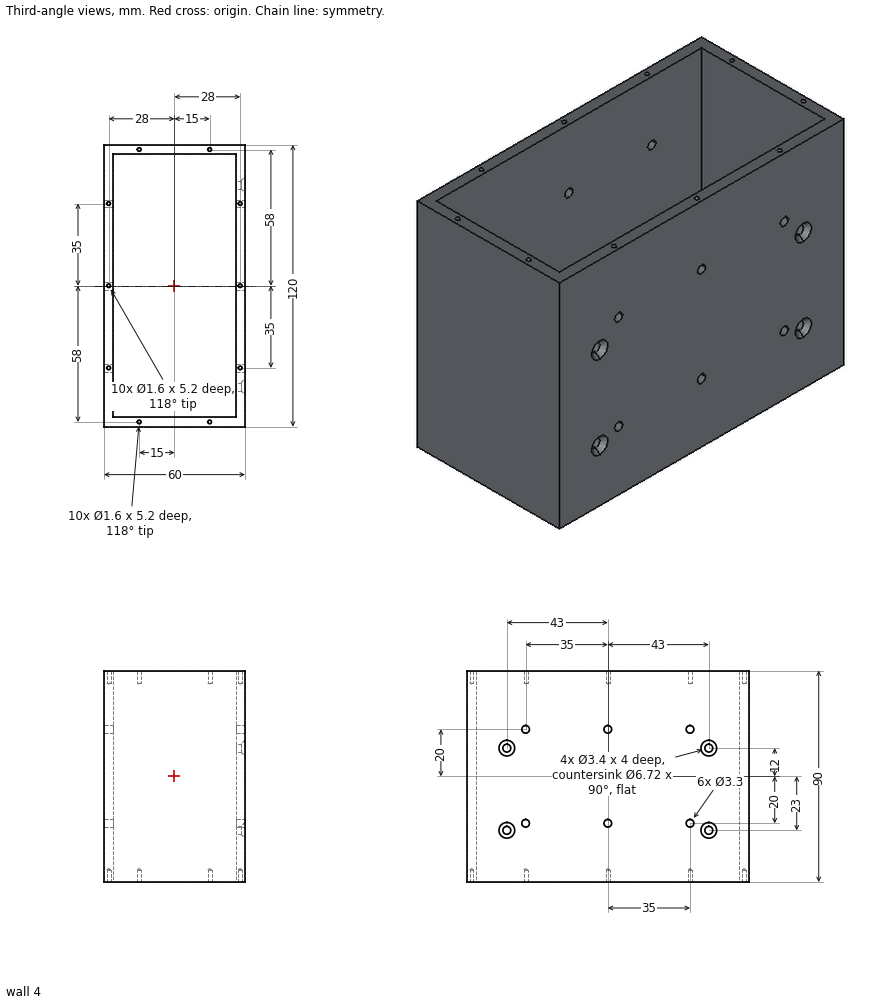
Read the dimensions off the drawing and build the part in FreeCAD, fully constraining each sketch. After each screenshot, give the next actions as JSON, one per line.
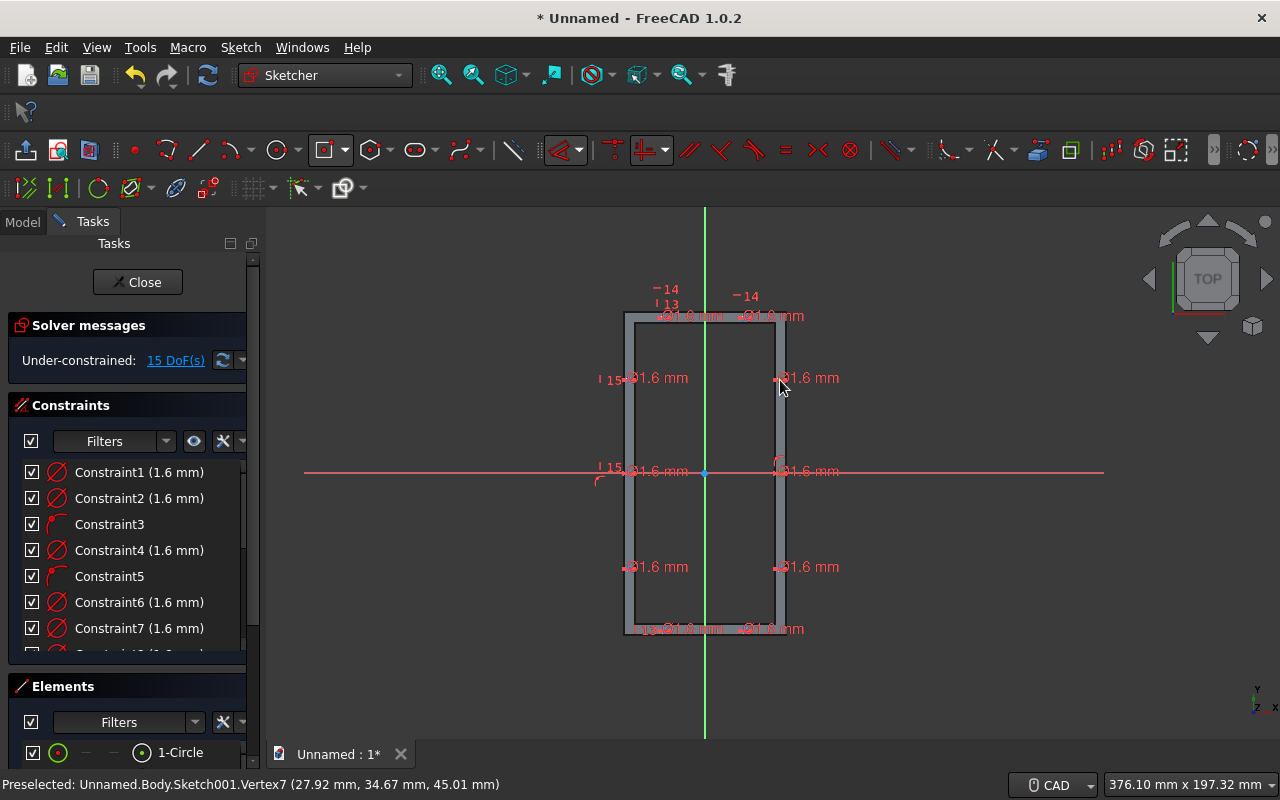
{"action": "left_click", "coordinate": [668, 150]}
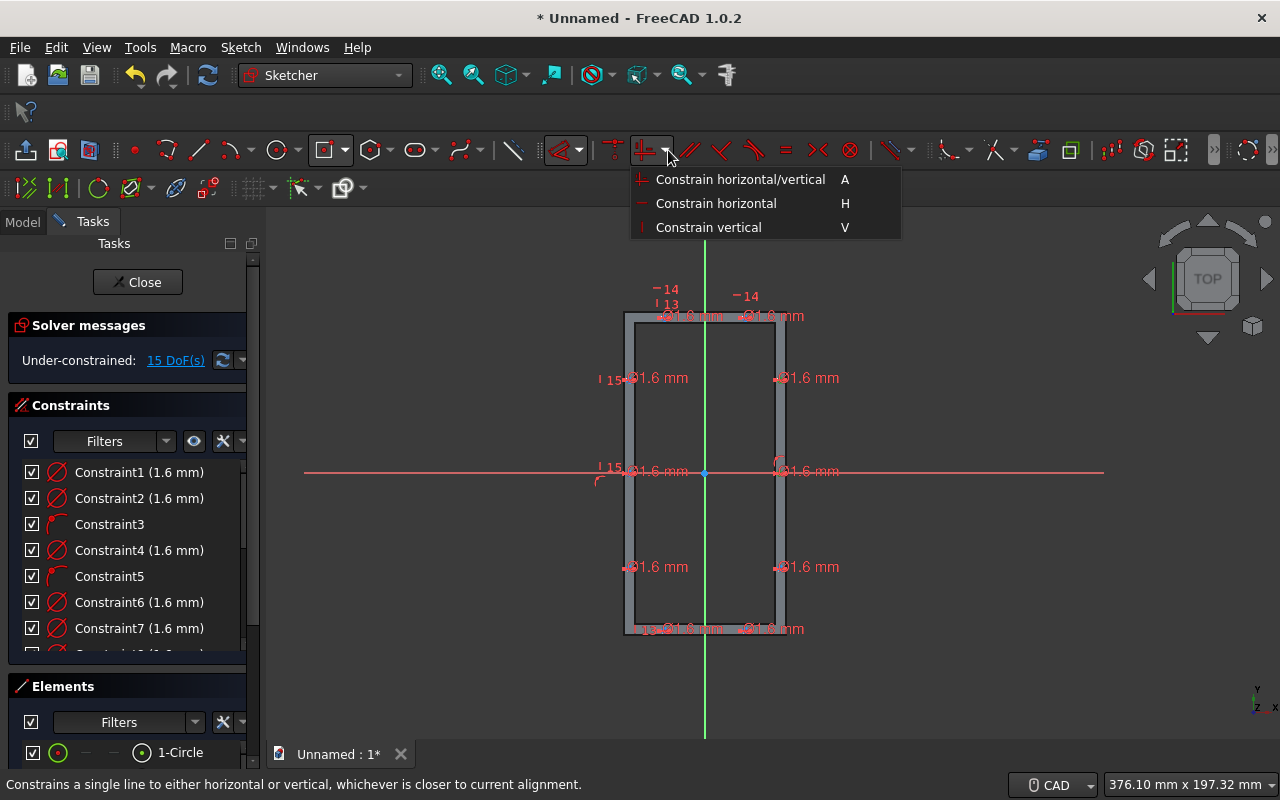
{"action": "left_click", "coordinate": [766, 227]}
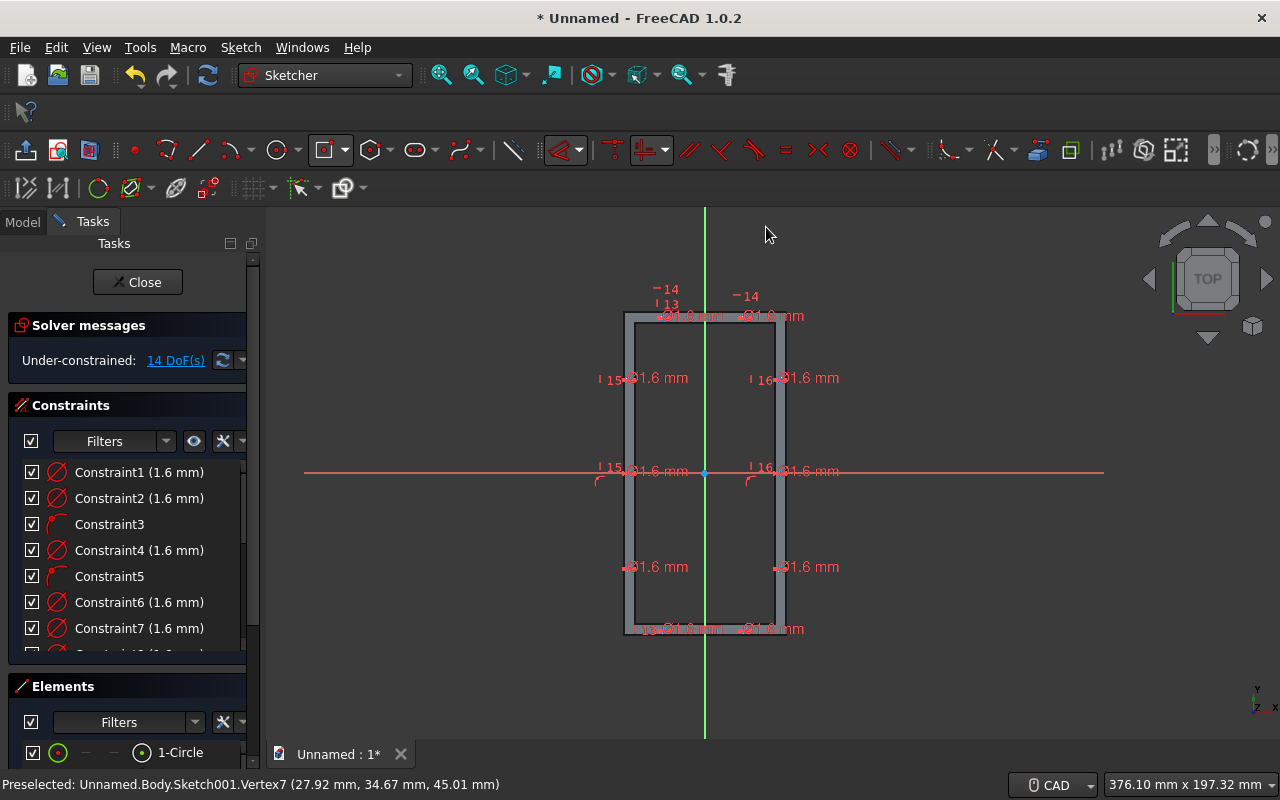
{"action": "left_click", "coordinate": [629, 380]}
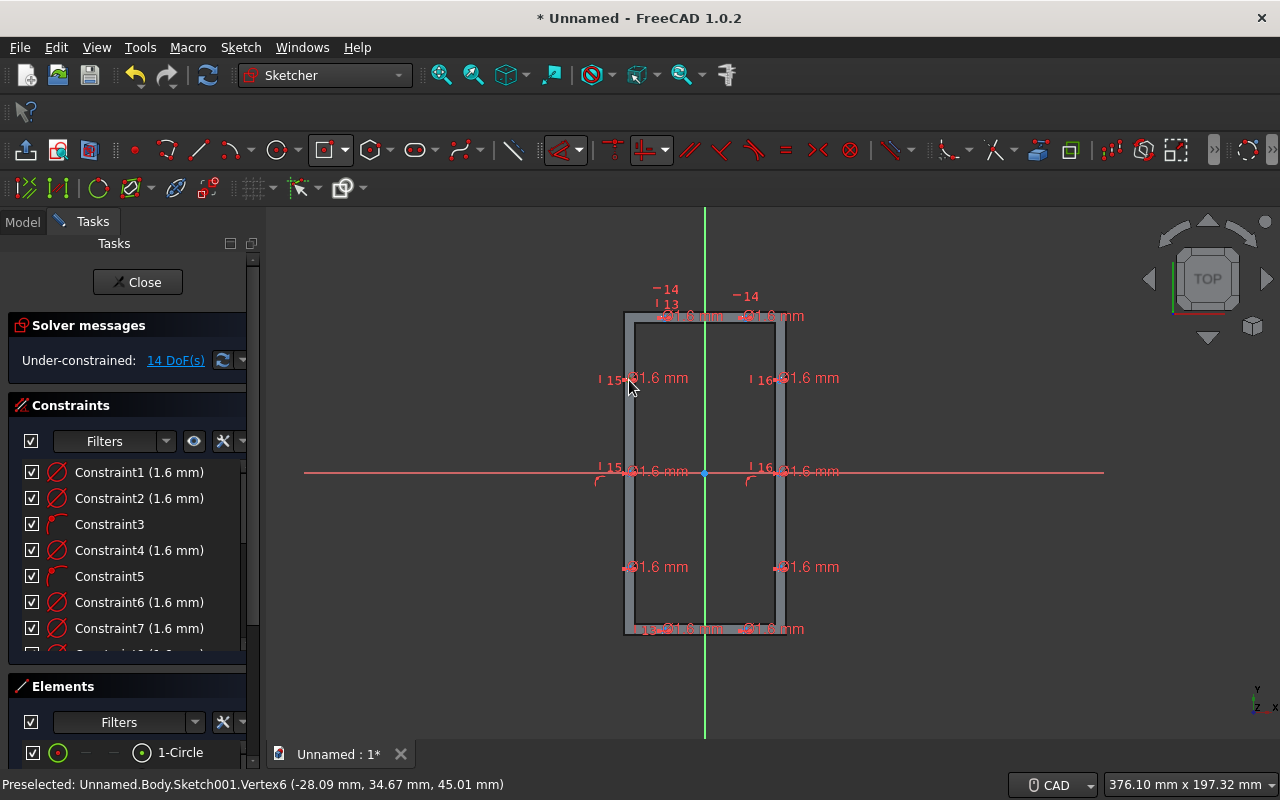
{"action": "left_click", "coordinate": [780, 380]}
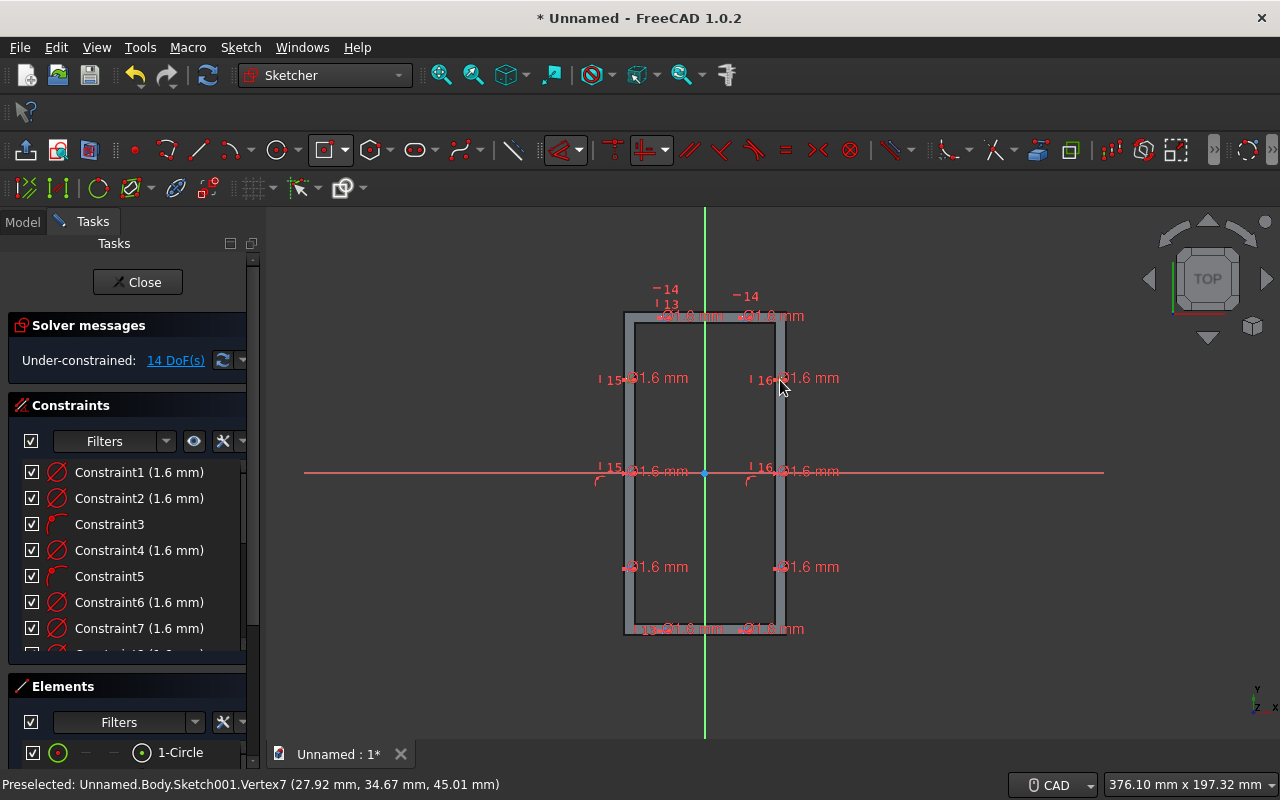
{"action": "left_click", "coordinate": [668, 150]}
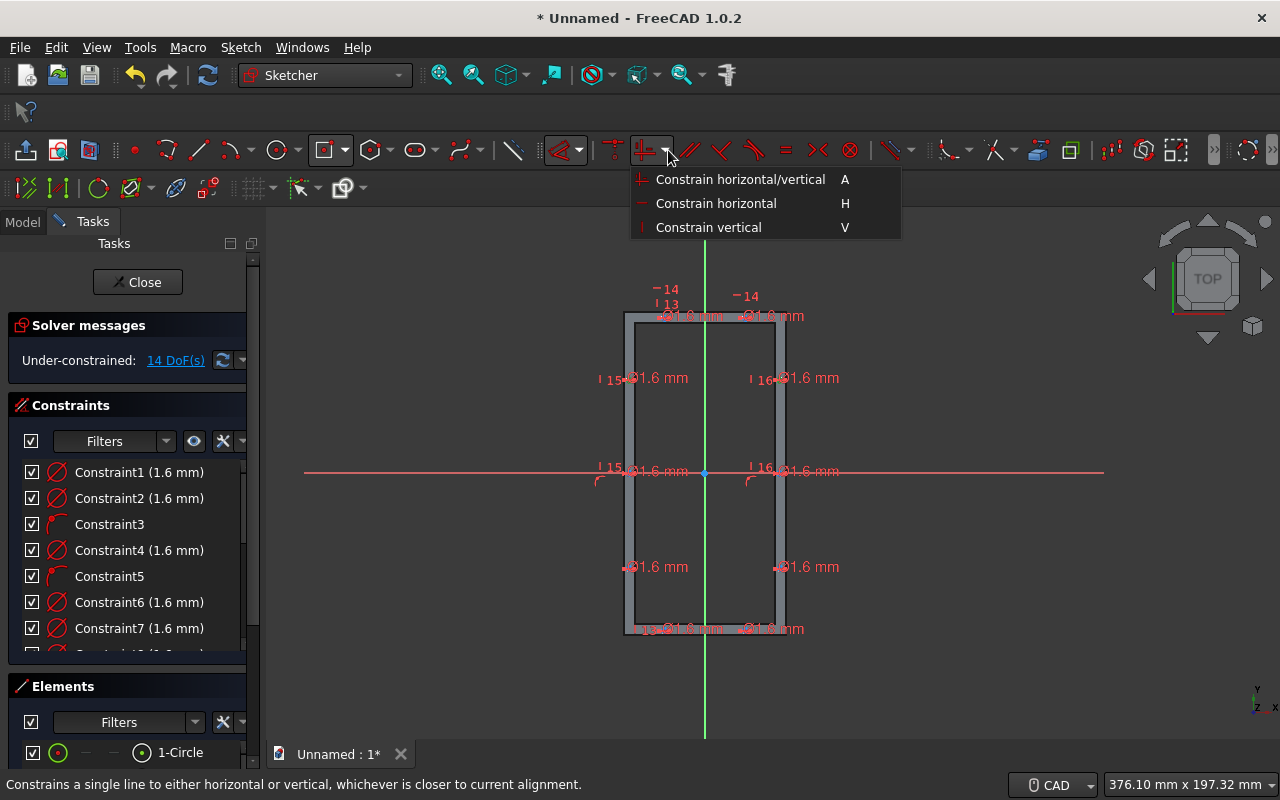
{"action": "left_click", "coordinate": [766, 203]}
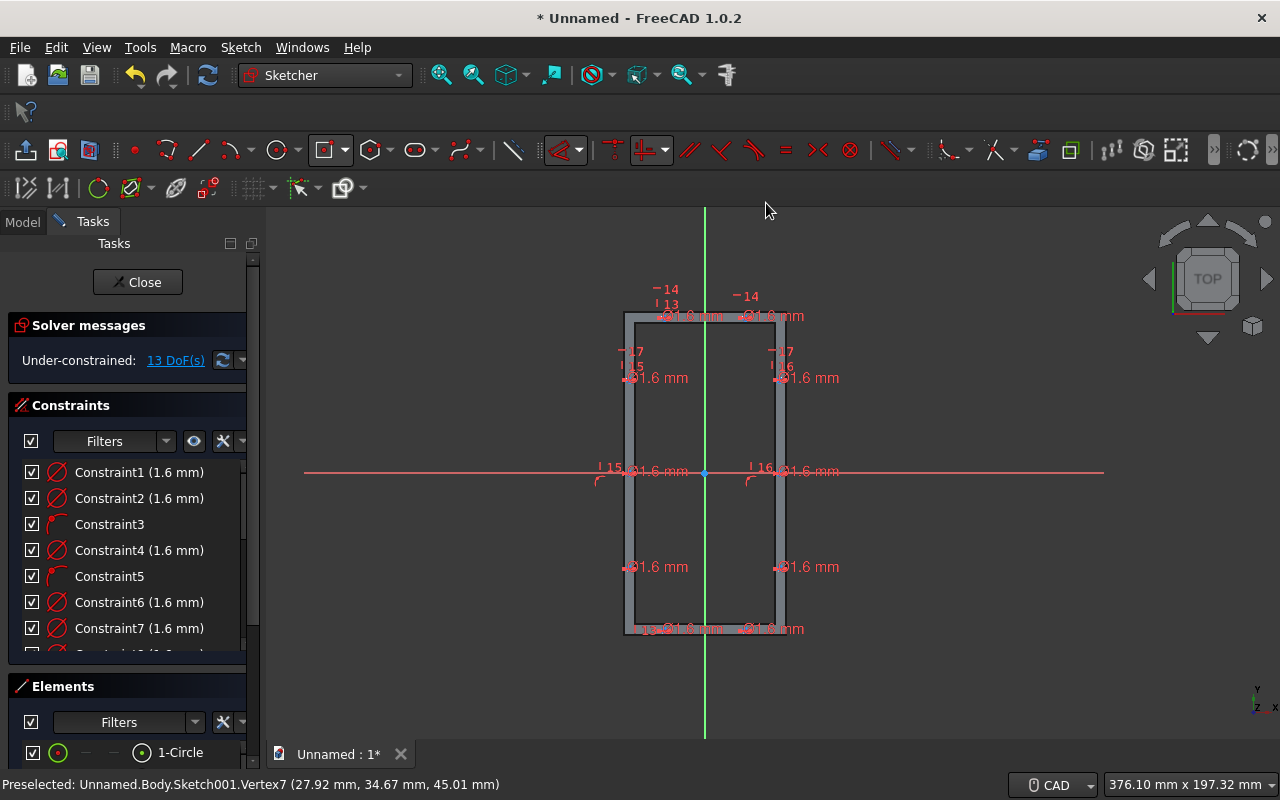
{"action": "left_click", "coordinate": [780, 473]}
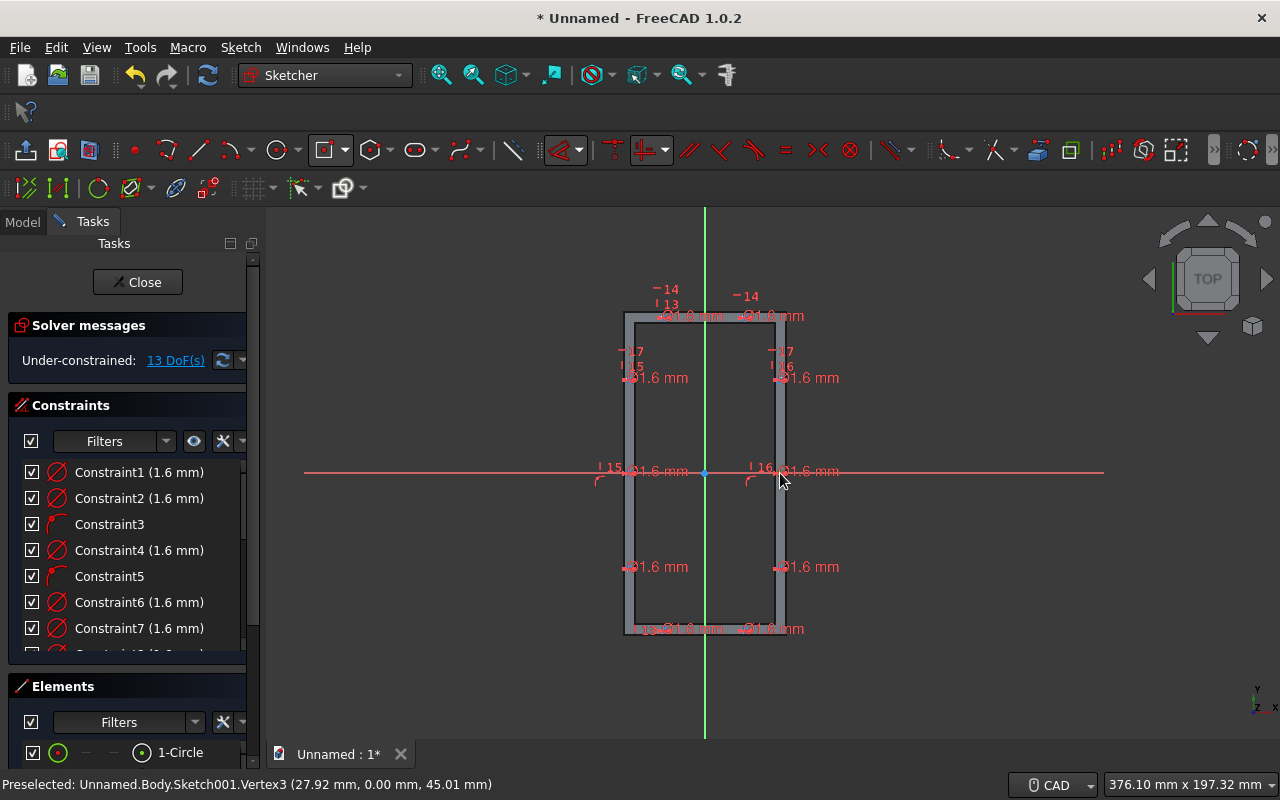
{"action": "left_click", "coordinate": [780, 569]}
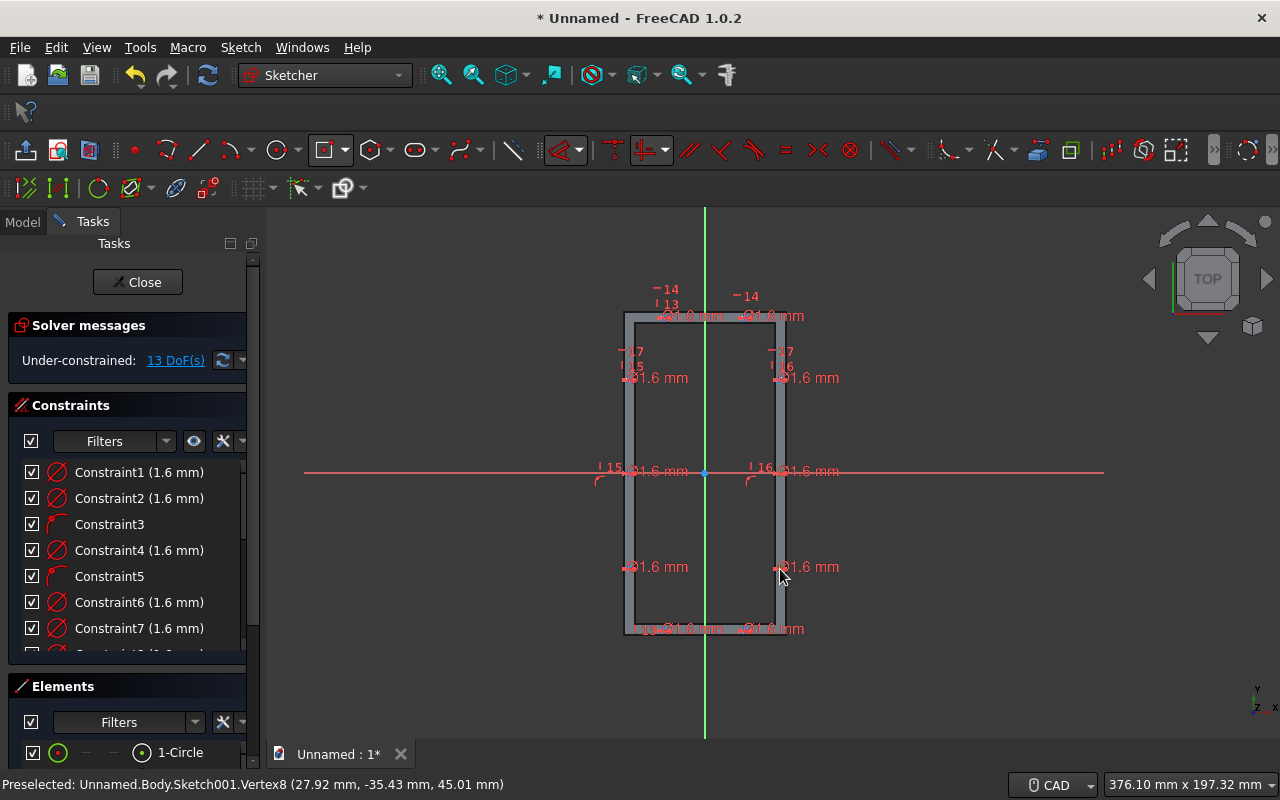
{"action": "key", "text": "v"}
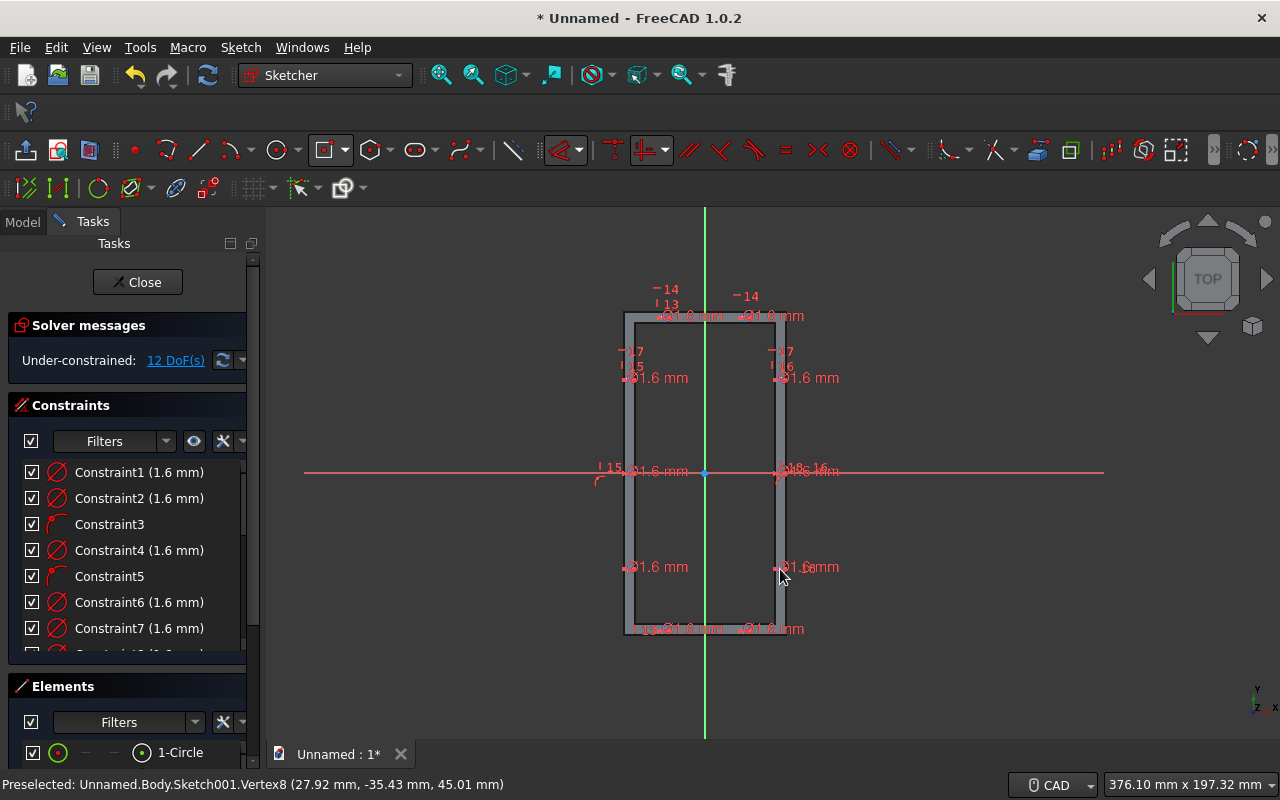
{"action": "left_click", "coordinate": [629, 473]}